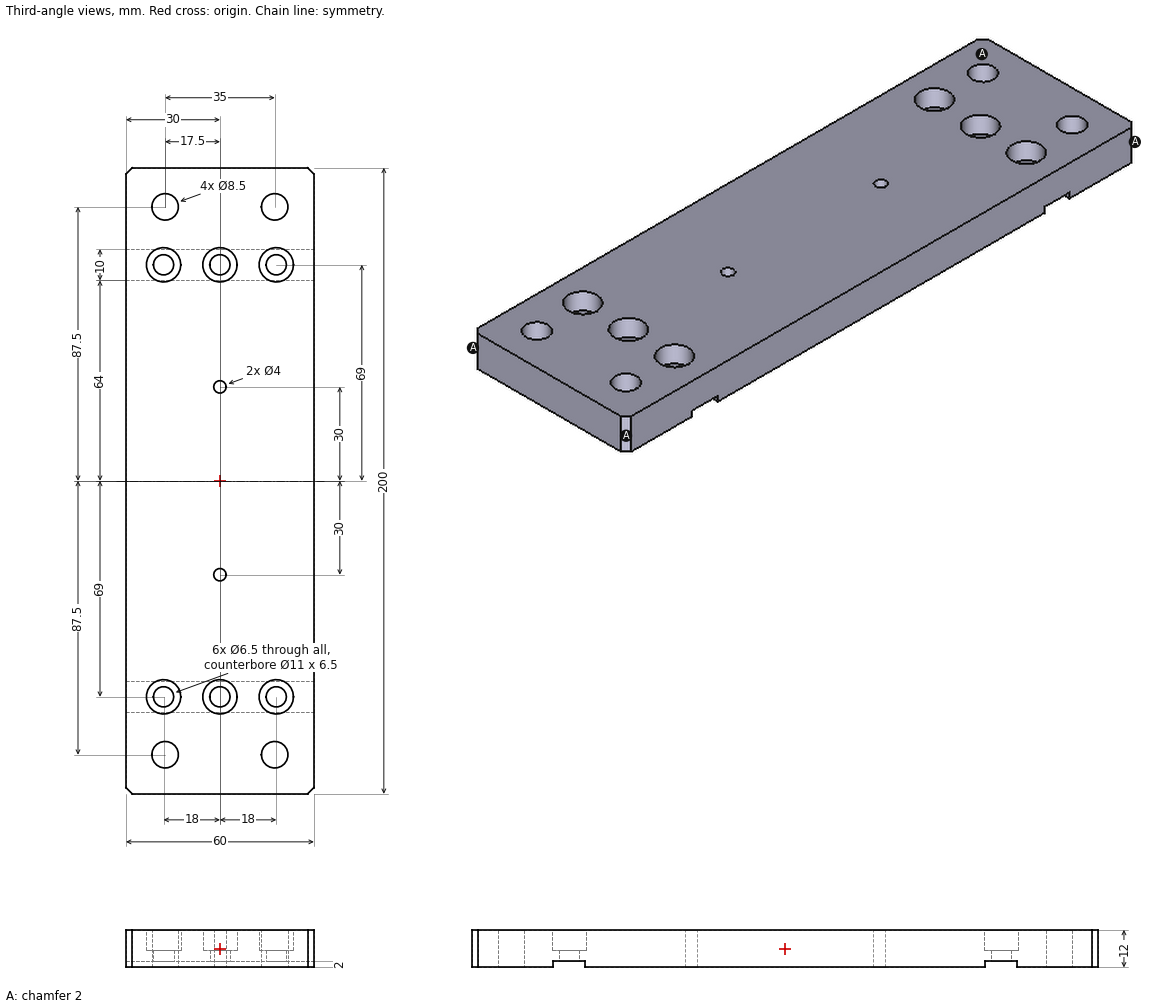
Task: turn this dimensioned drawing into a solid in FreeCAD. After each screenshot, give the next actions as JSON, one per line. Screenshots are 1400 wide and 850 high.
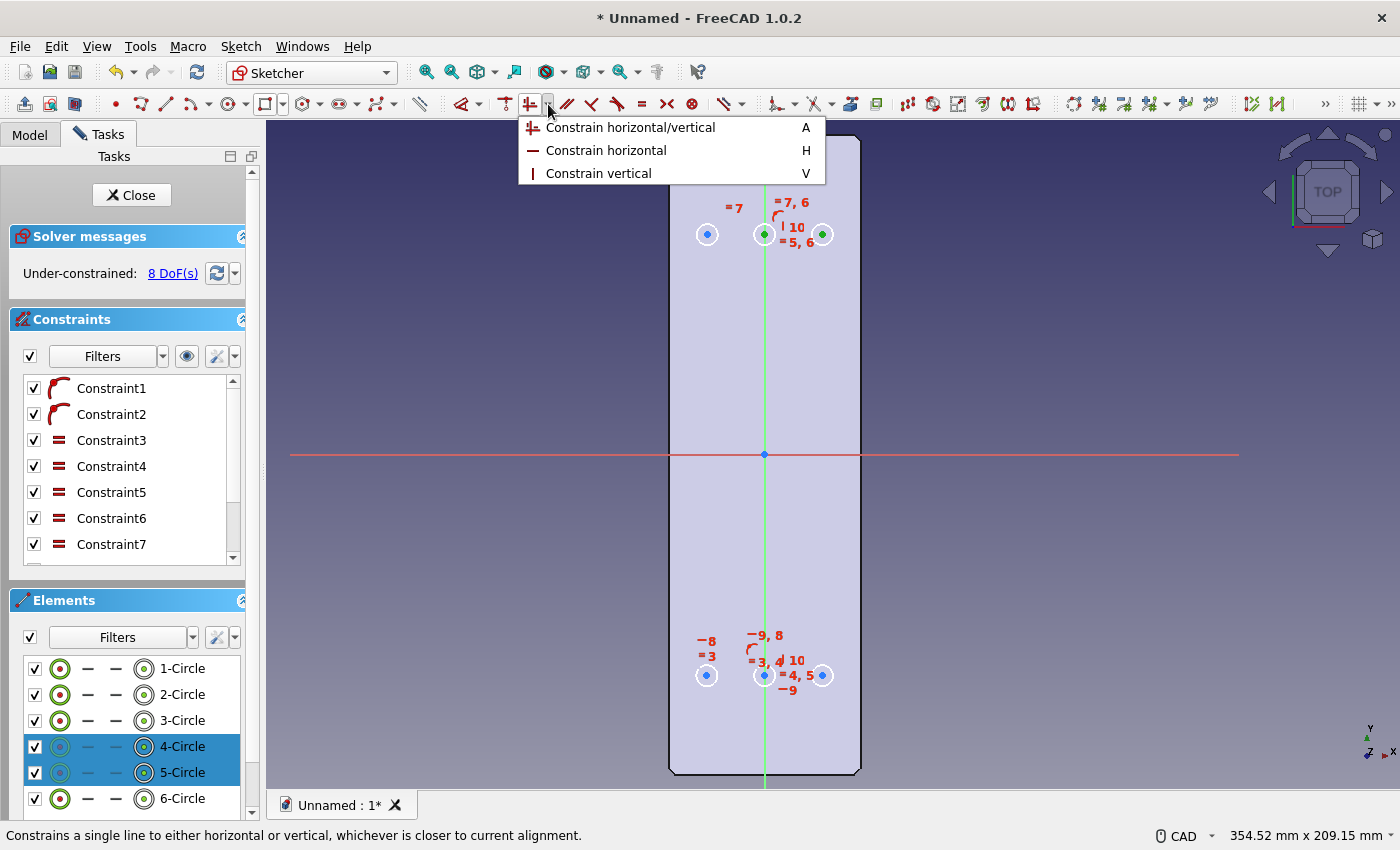
{"action": "left_click", "coordinate": [672, 150]}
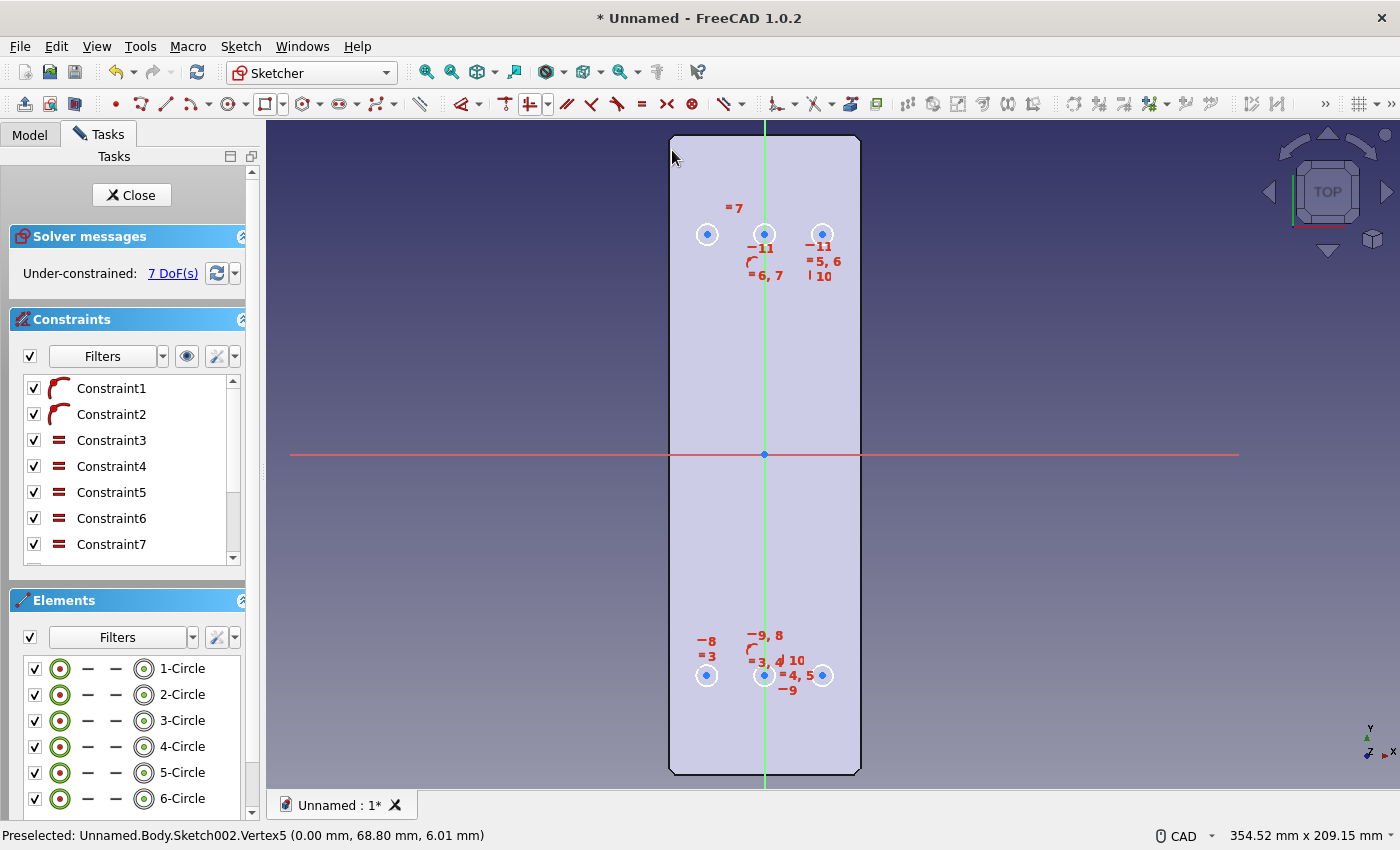
{"action": "left_click", "coordinate": [707, 676]}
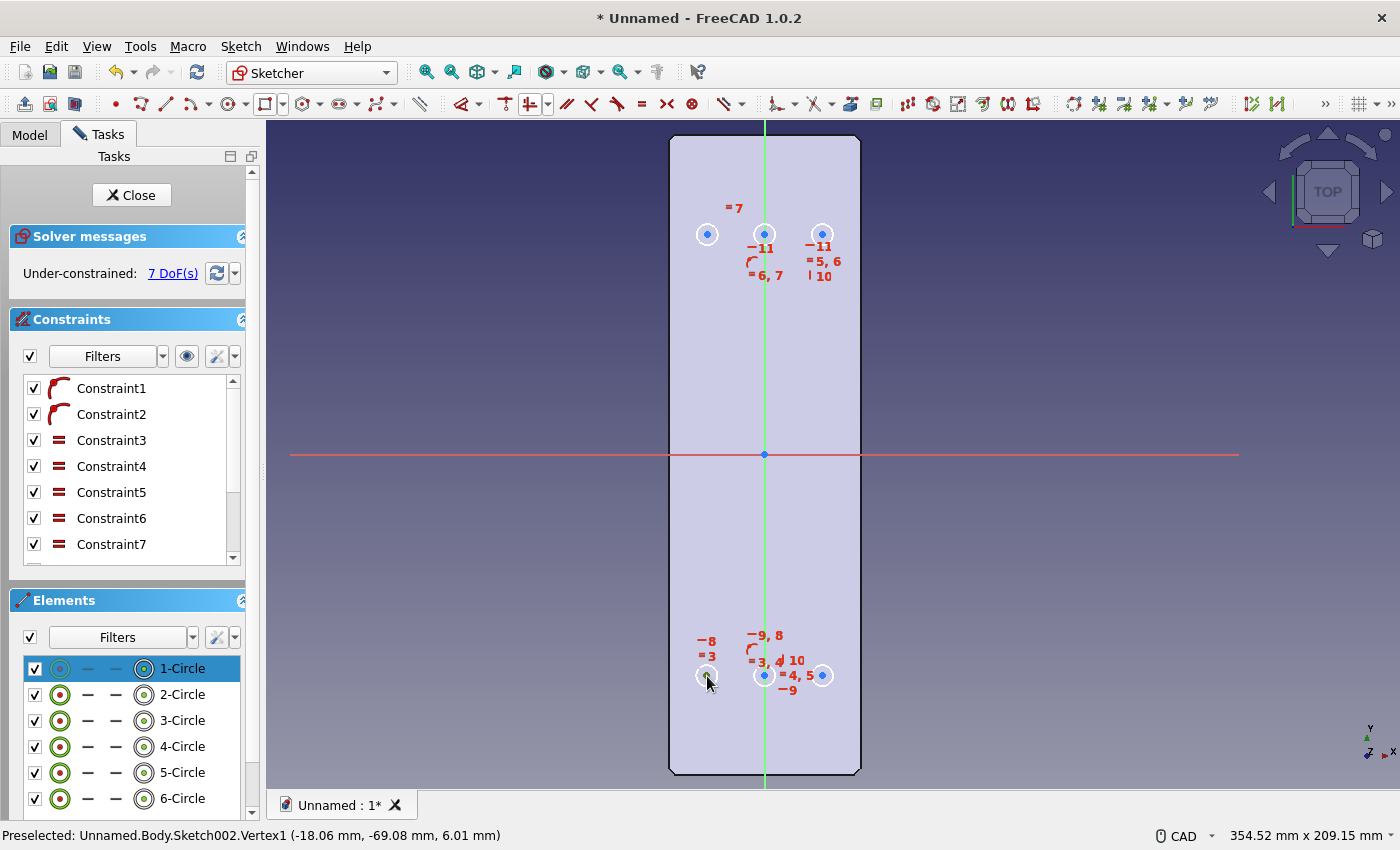
{"action": "left_click", "coordinate": [707, 235]}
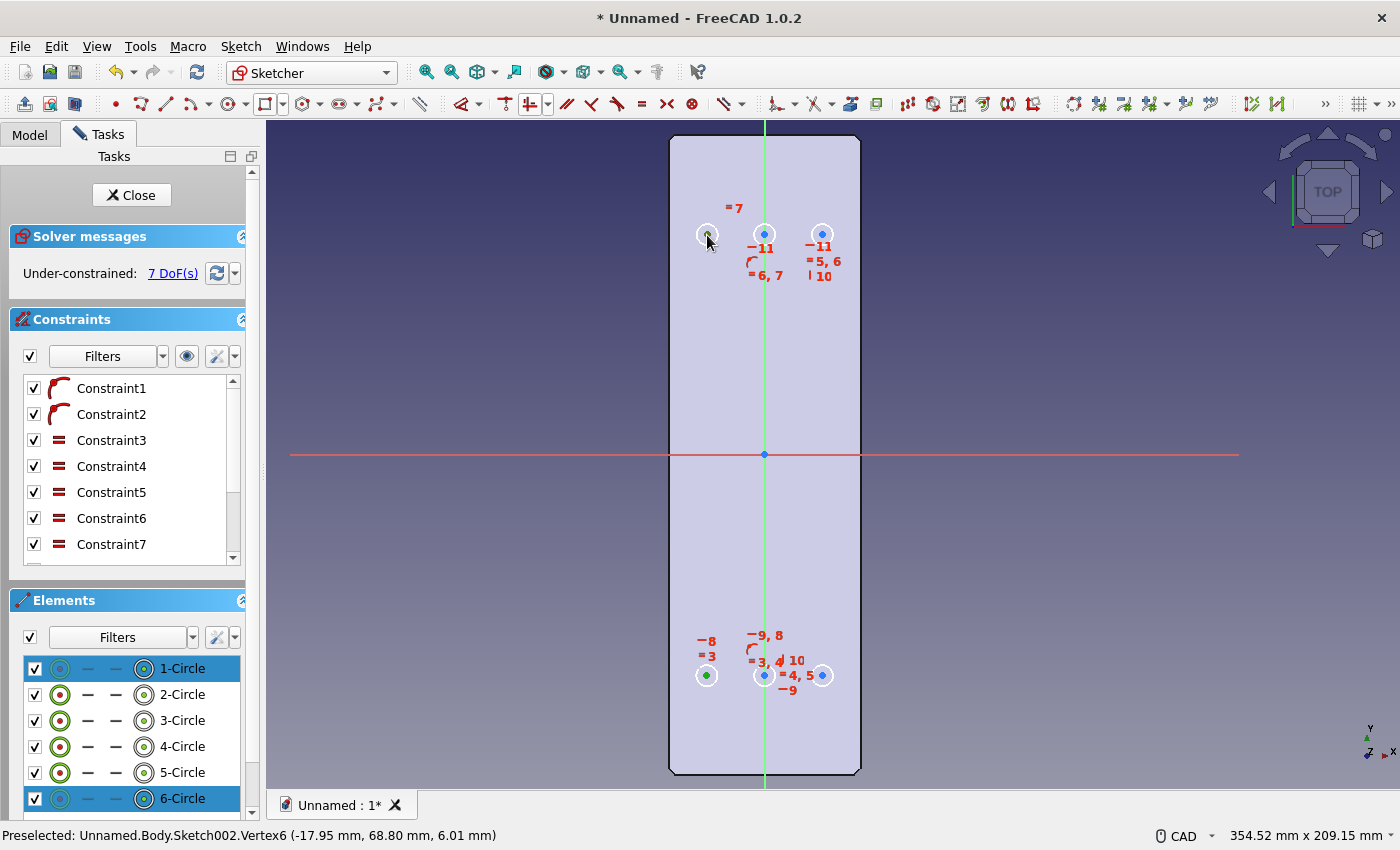
{"action": "left_click", "coordinate": [548, 104]}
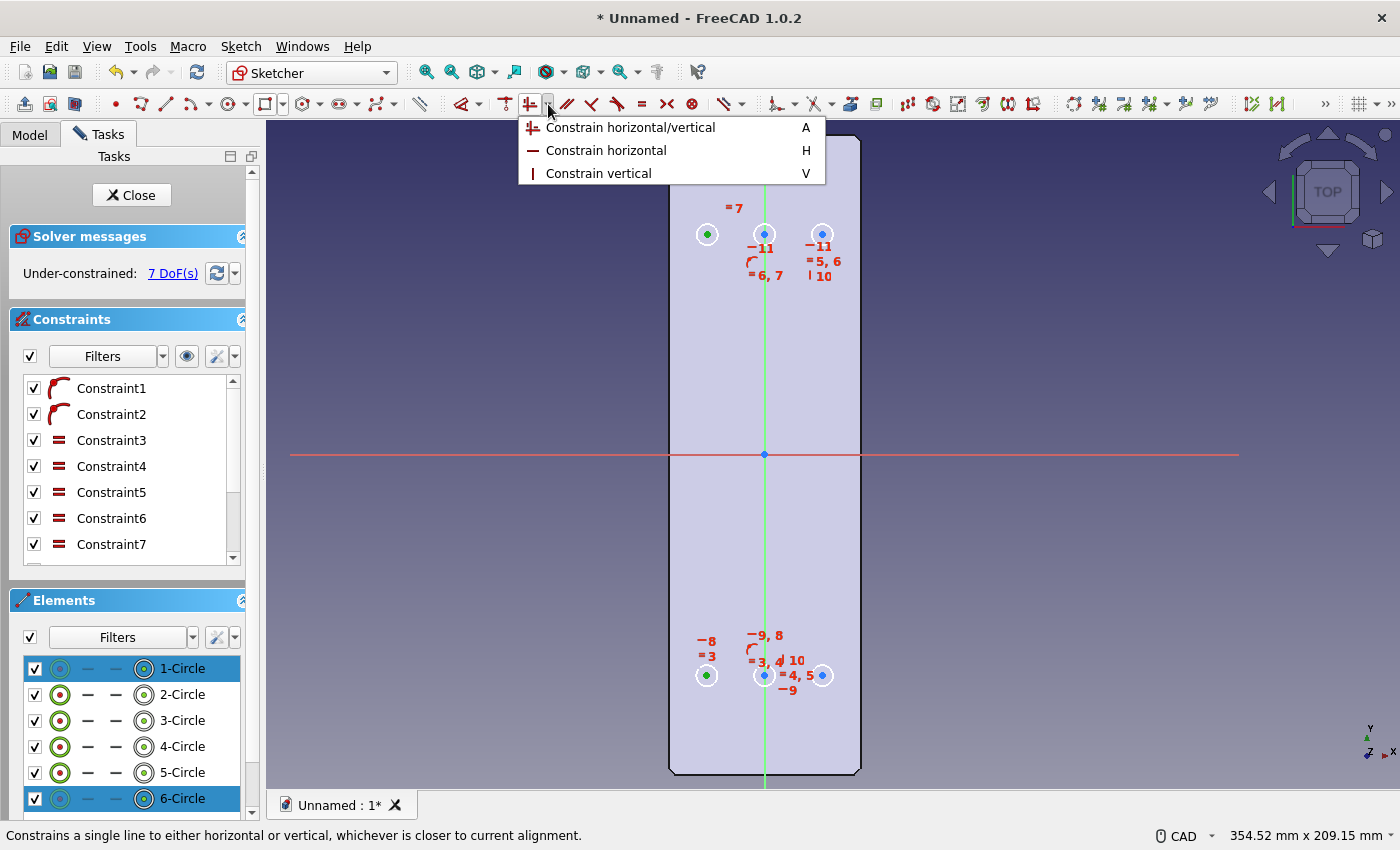
{"action": "left_click", "coordinate": [672, 174]}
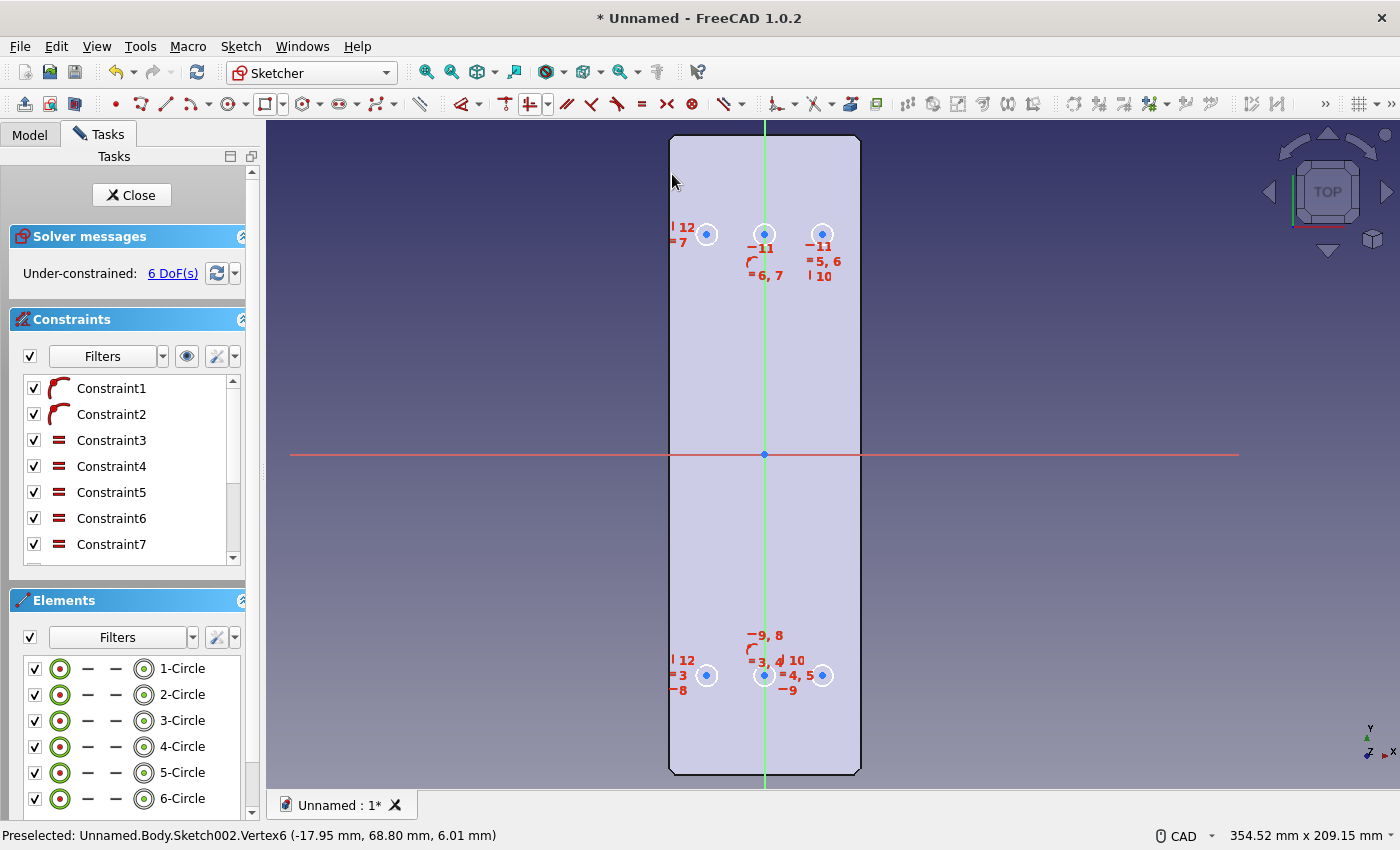
{"action": "left_click", "coordinate": [765, 235]}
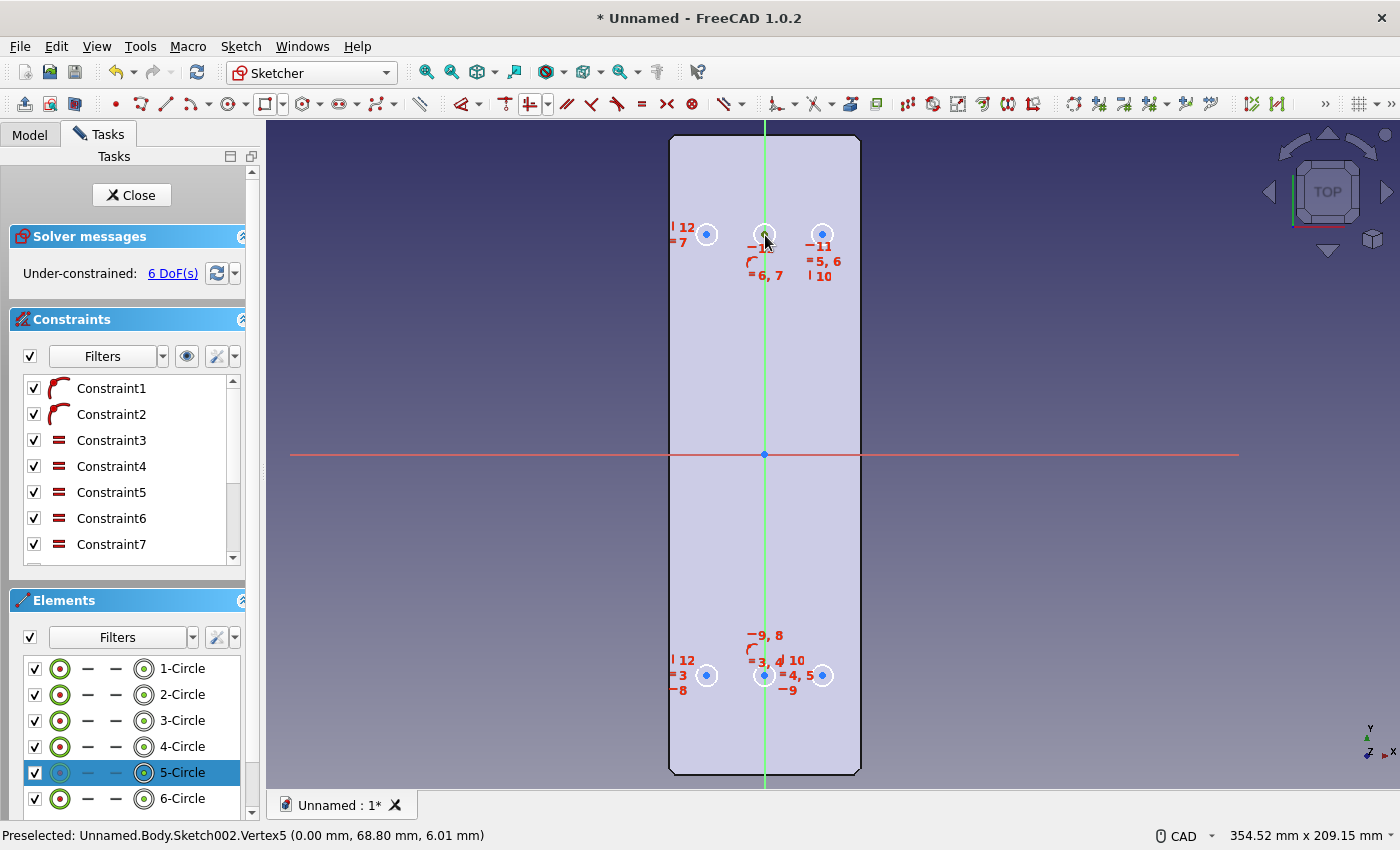
{"action": "left_click", "coordinate": [707, 235]}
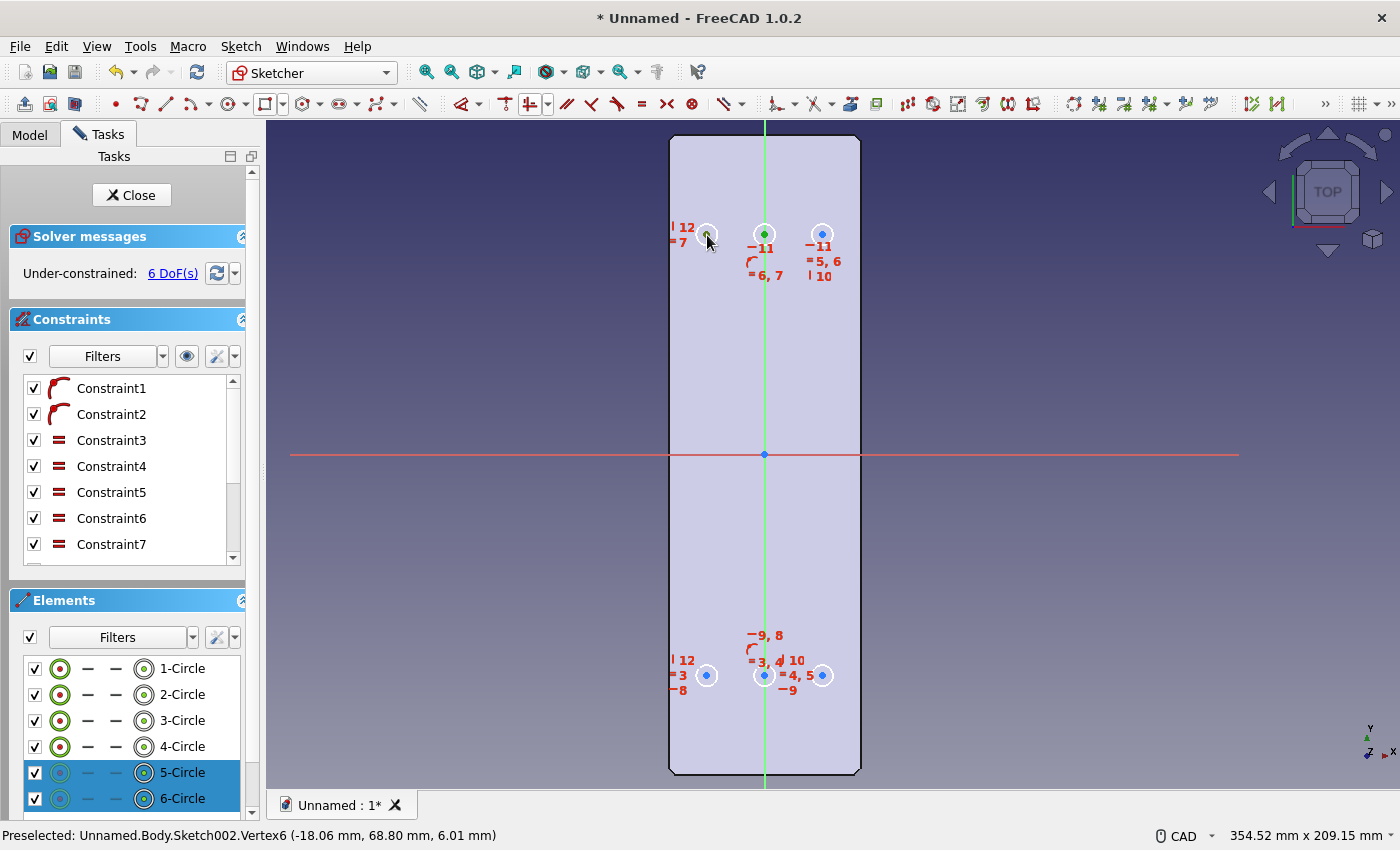
{"action": "left_click", "coordinate": [548, 104]}